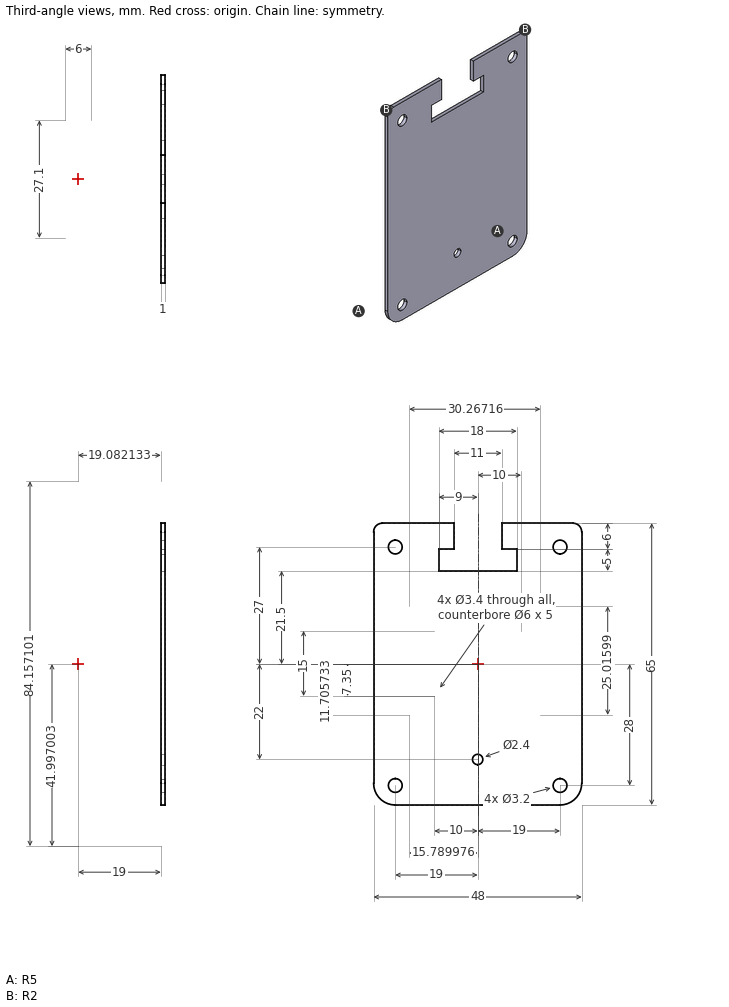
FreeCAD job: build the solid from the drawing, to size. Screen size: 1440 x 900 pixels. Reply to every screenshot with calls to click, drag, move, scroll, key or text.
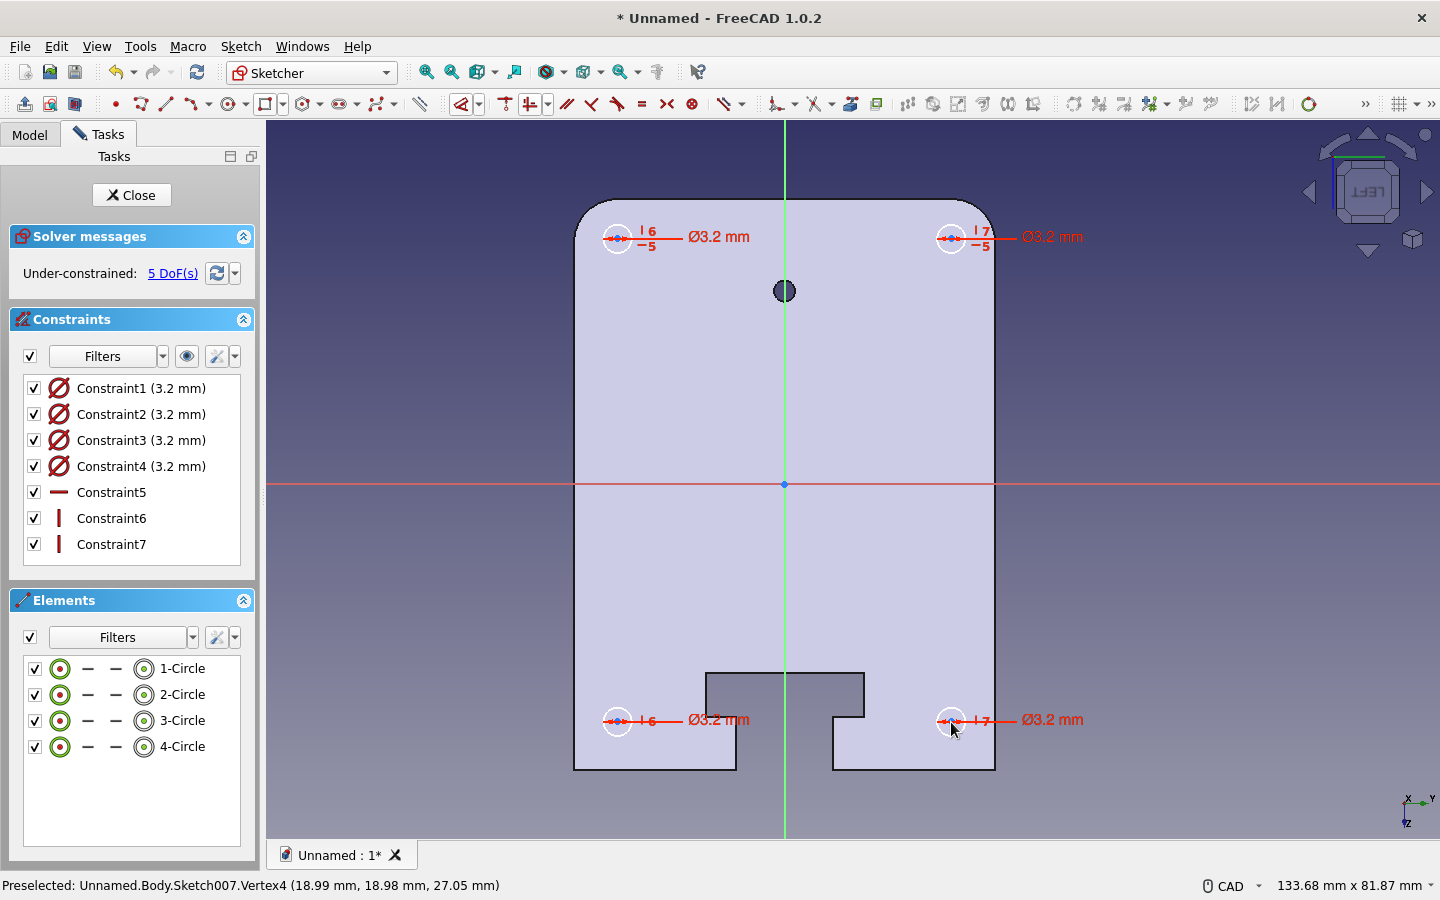
click(618, 722)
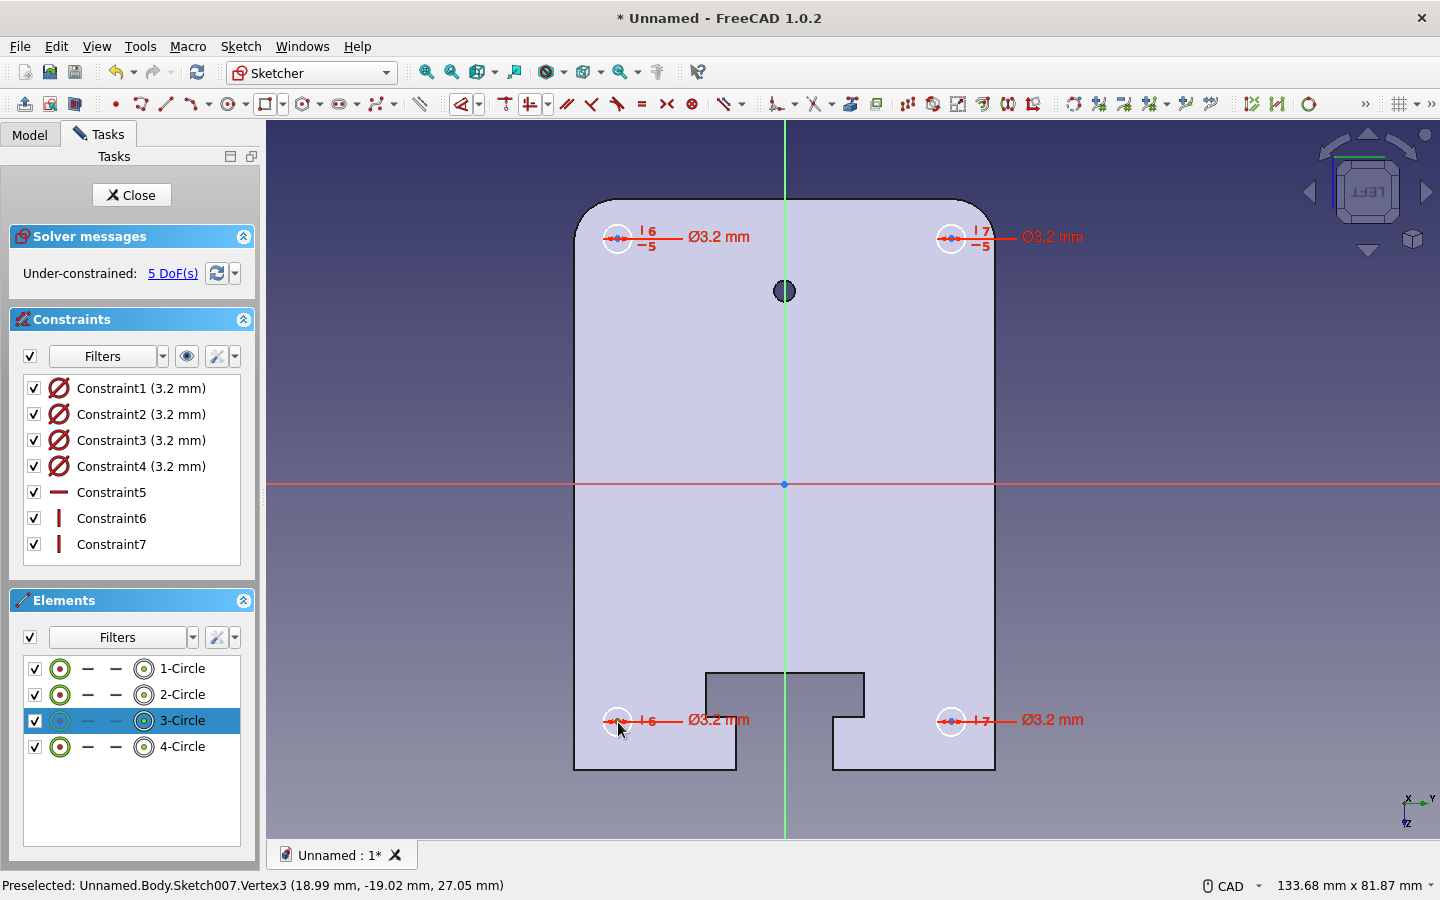
click(951, 722)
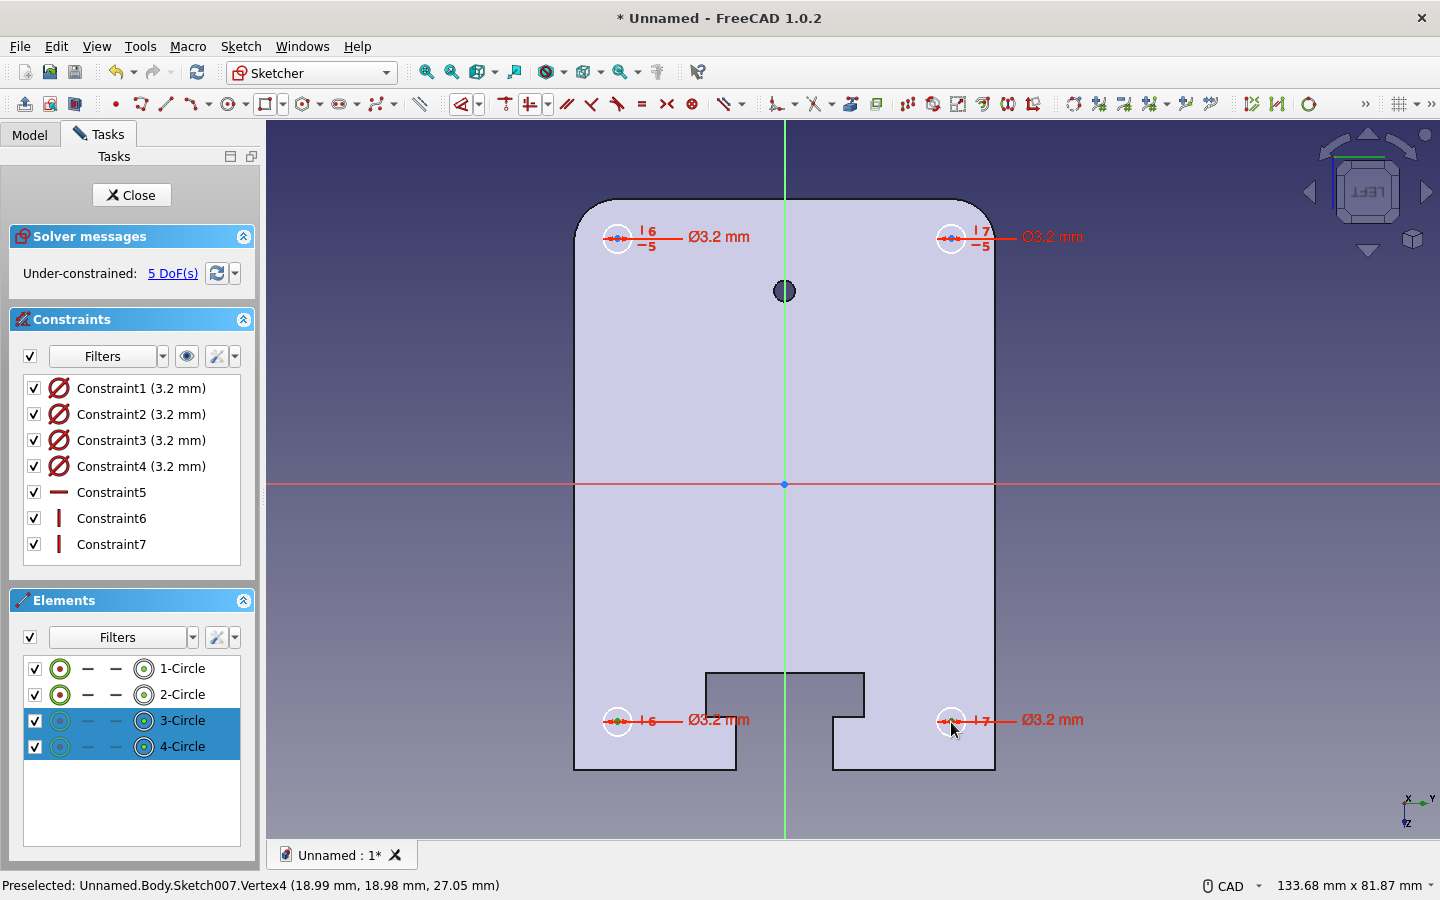
key(h)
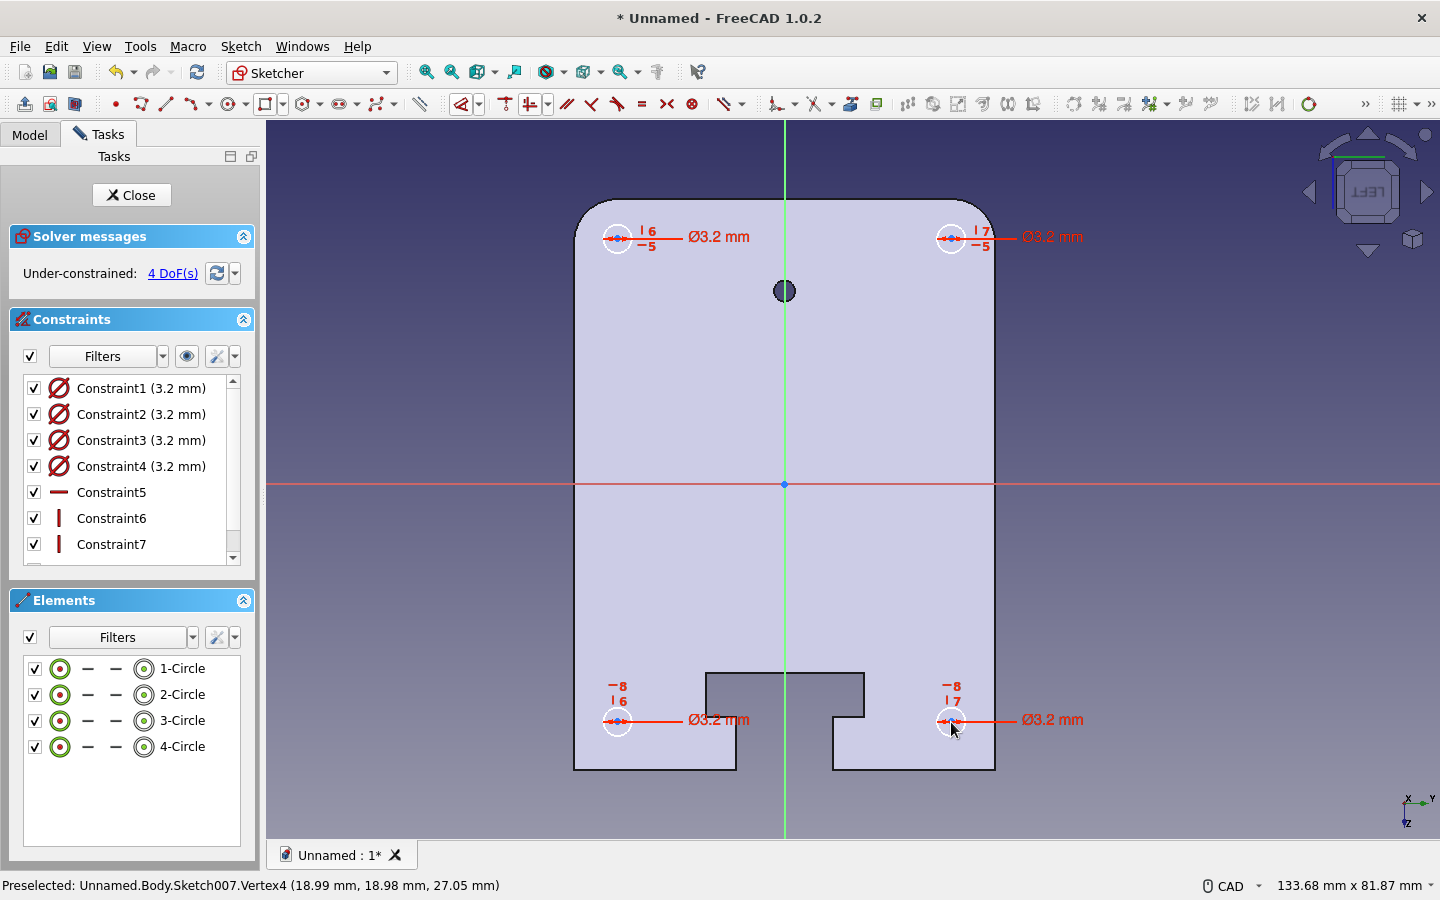
click(951, 239)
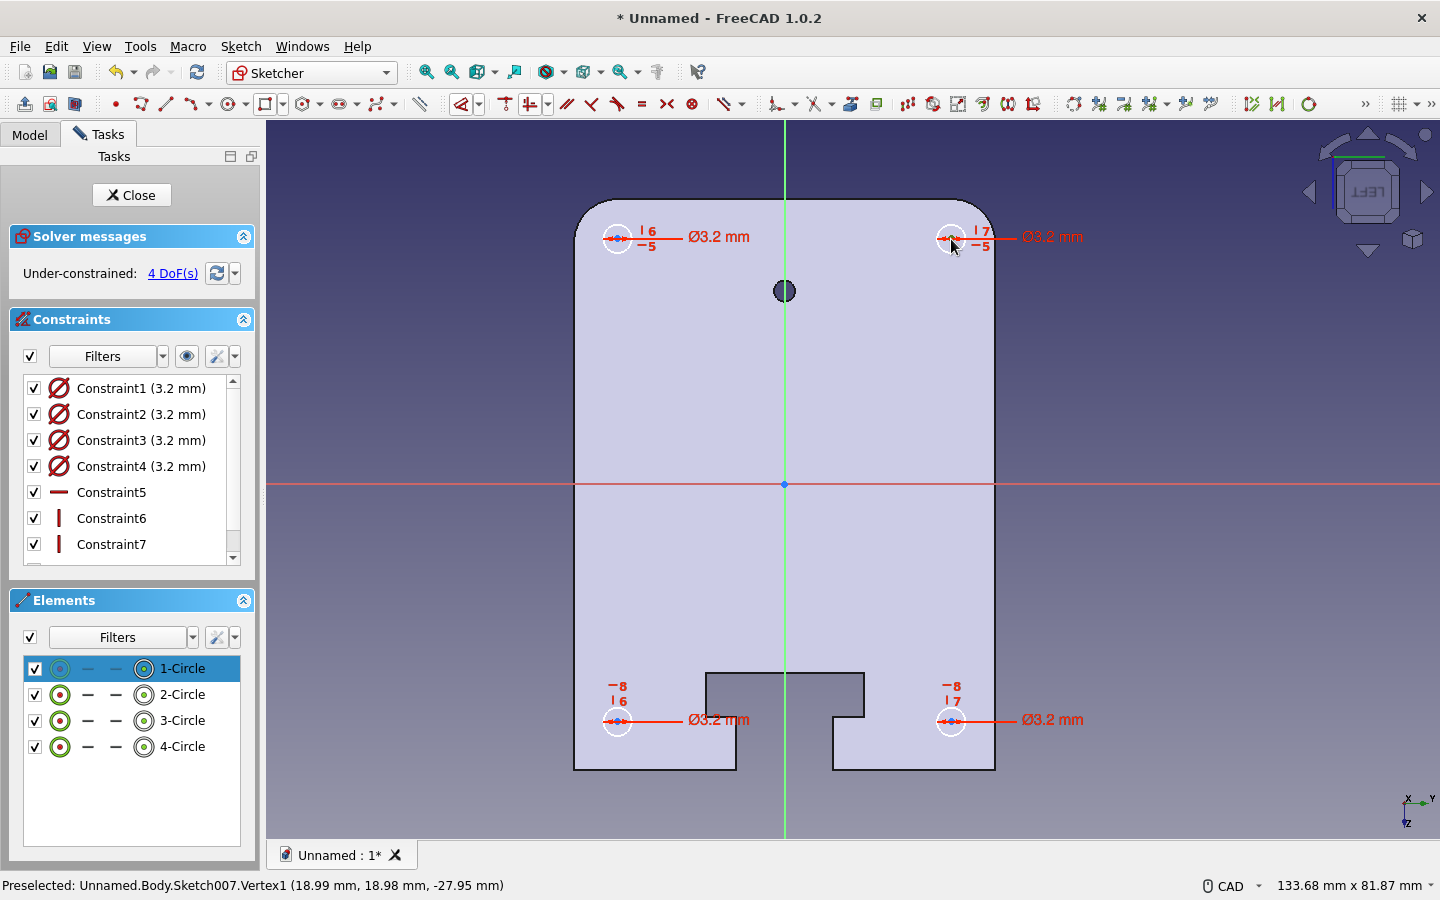
key(l)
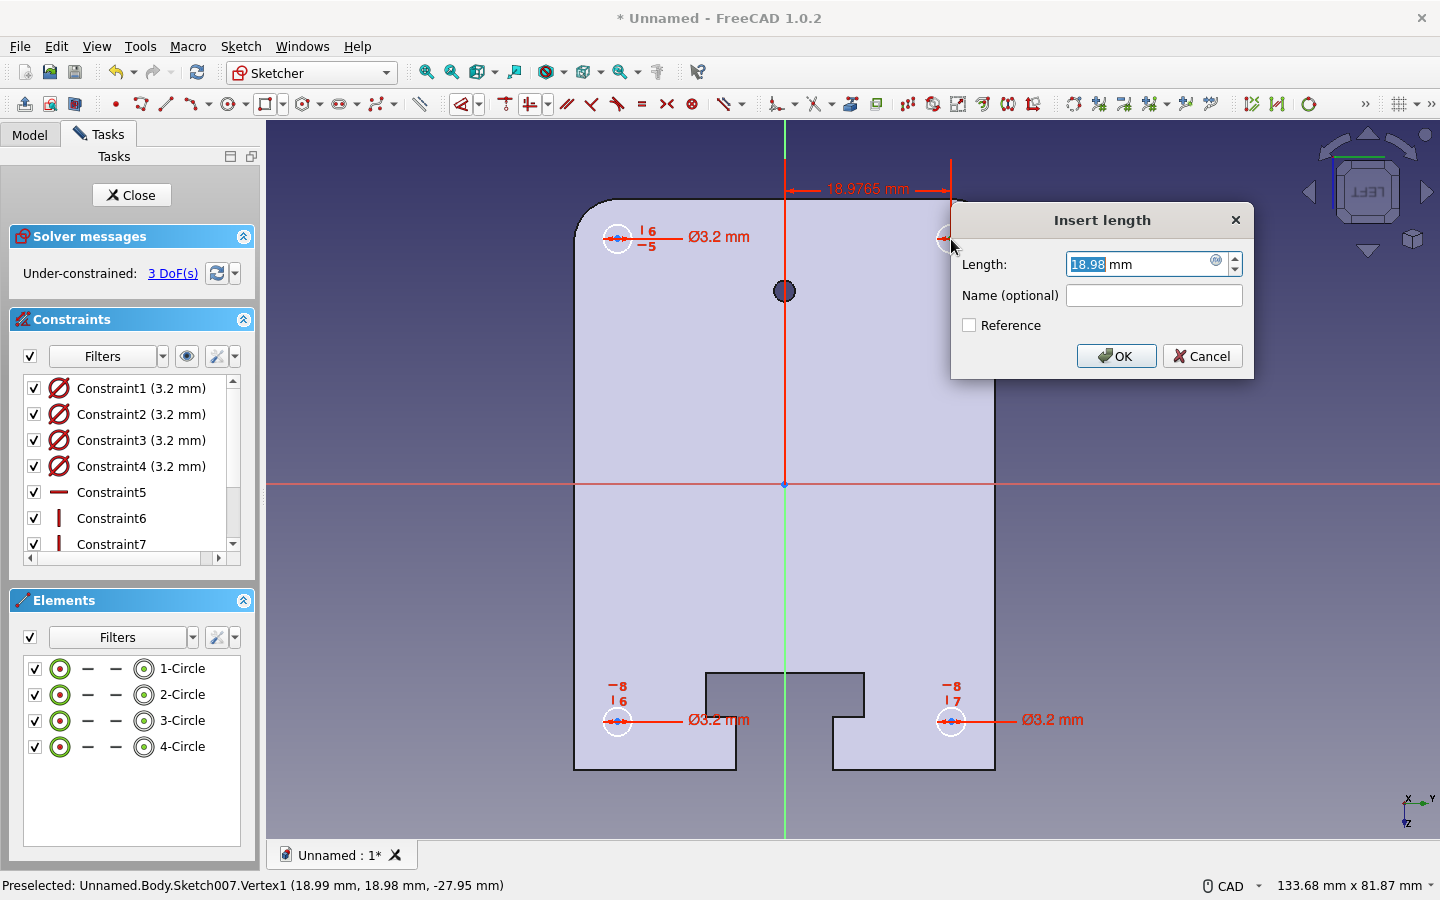
text(19)
key(Return)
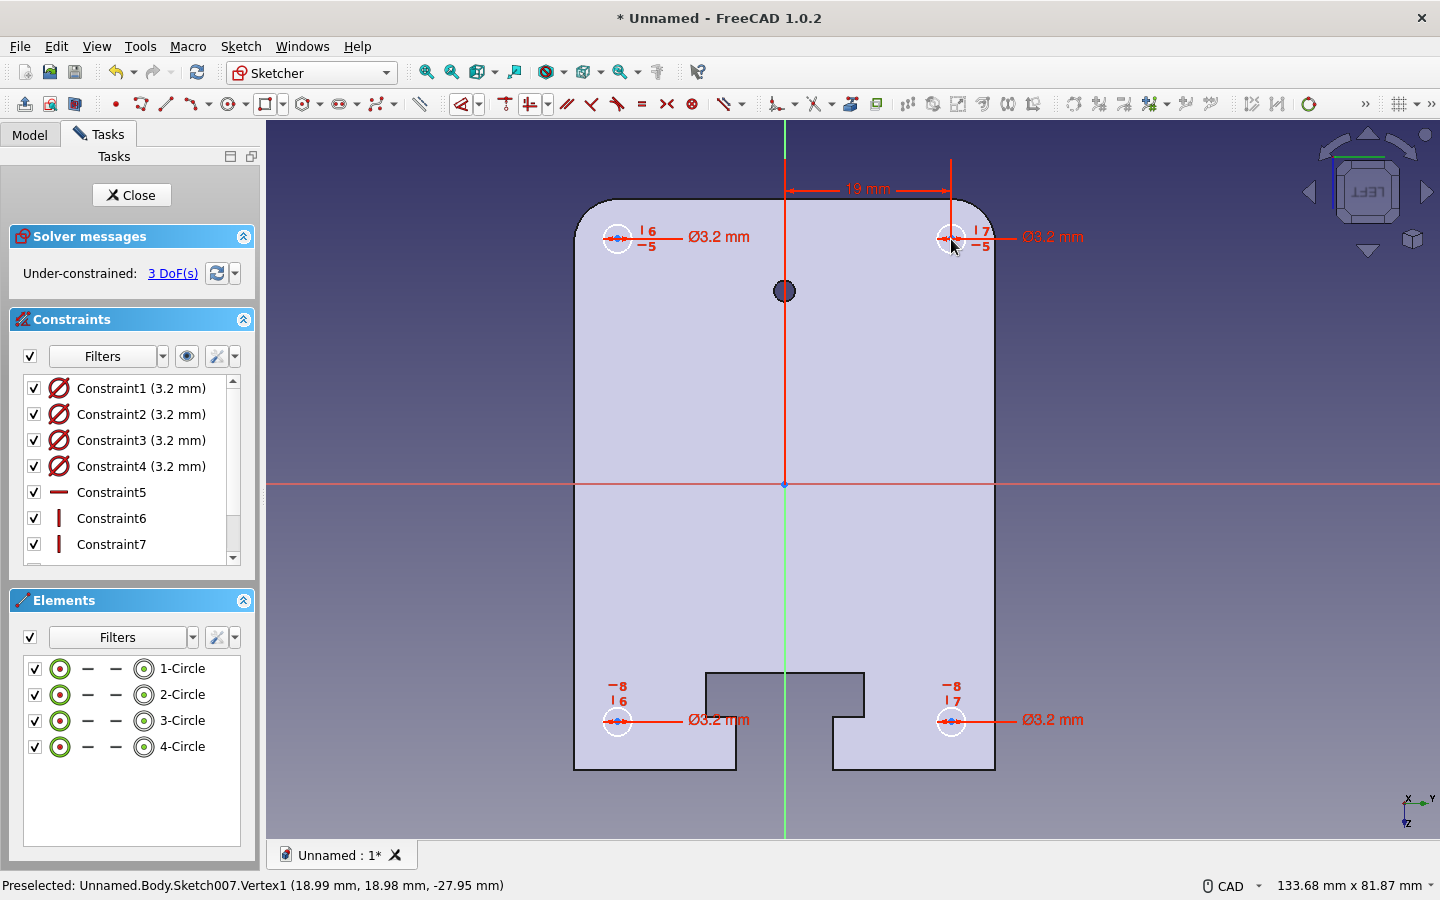
click(951, 239)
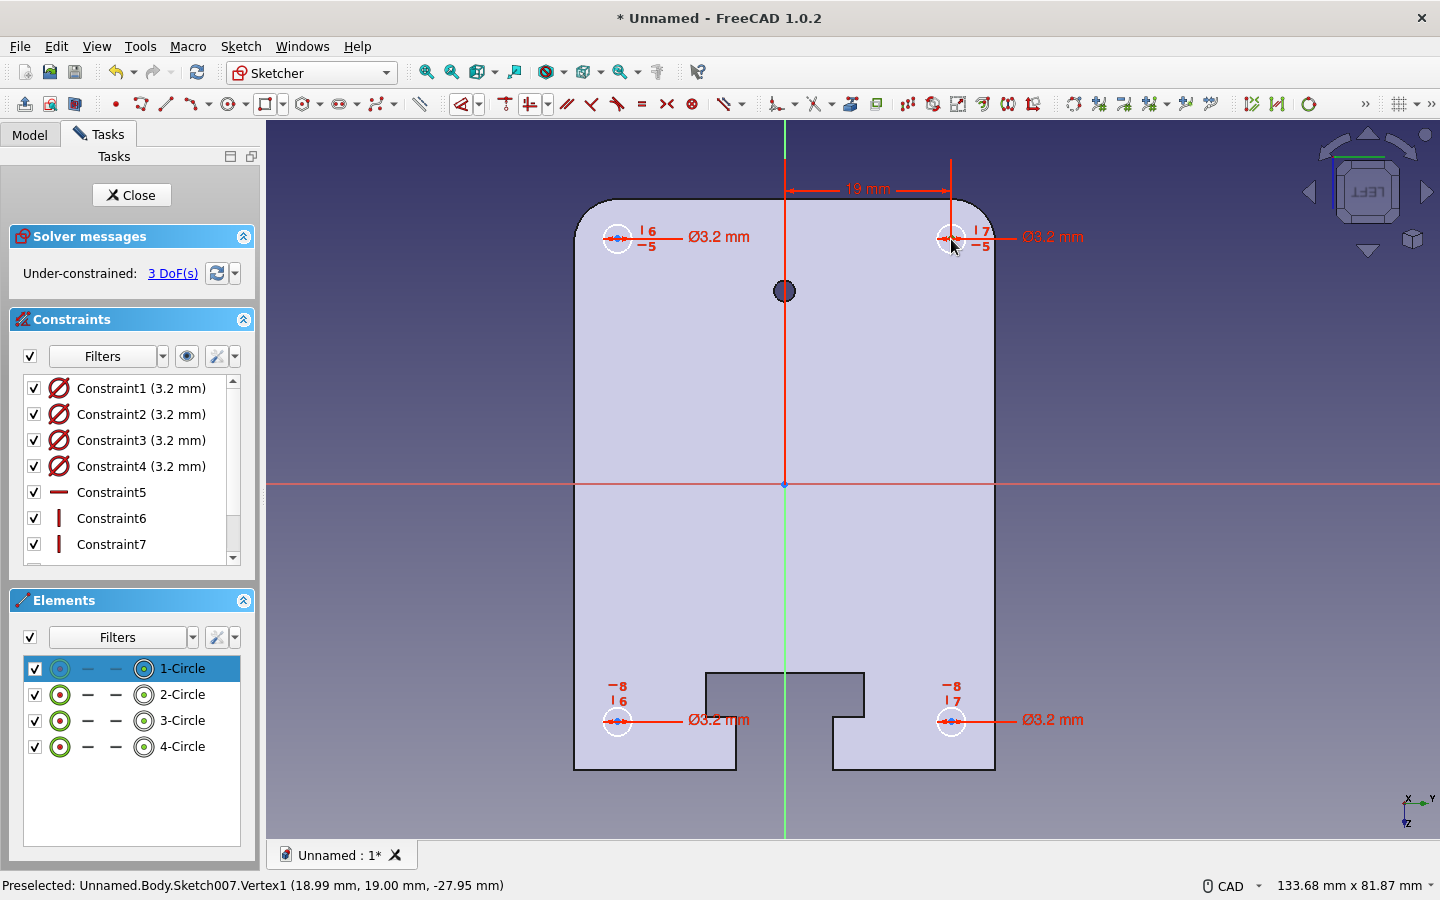
key(i)